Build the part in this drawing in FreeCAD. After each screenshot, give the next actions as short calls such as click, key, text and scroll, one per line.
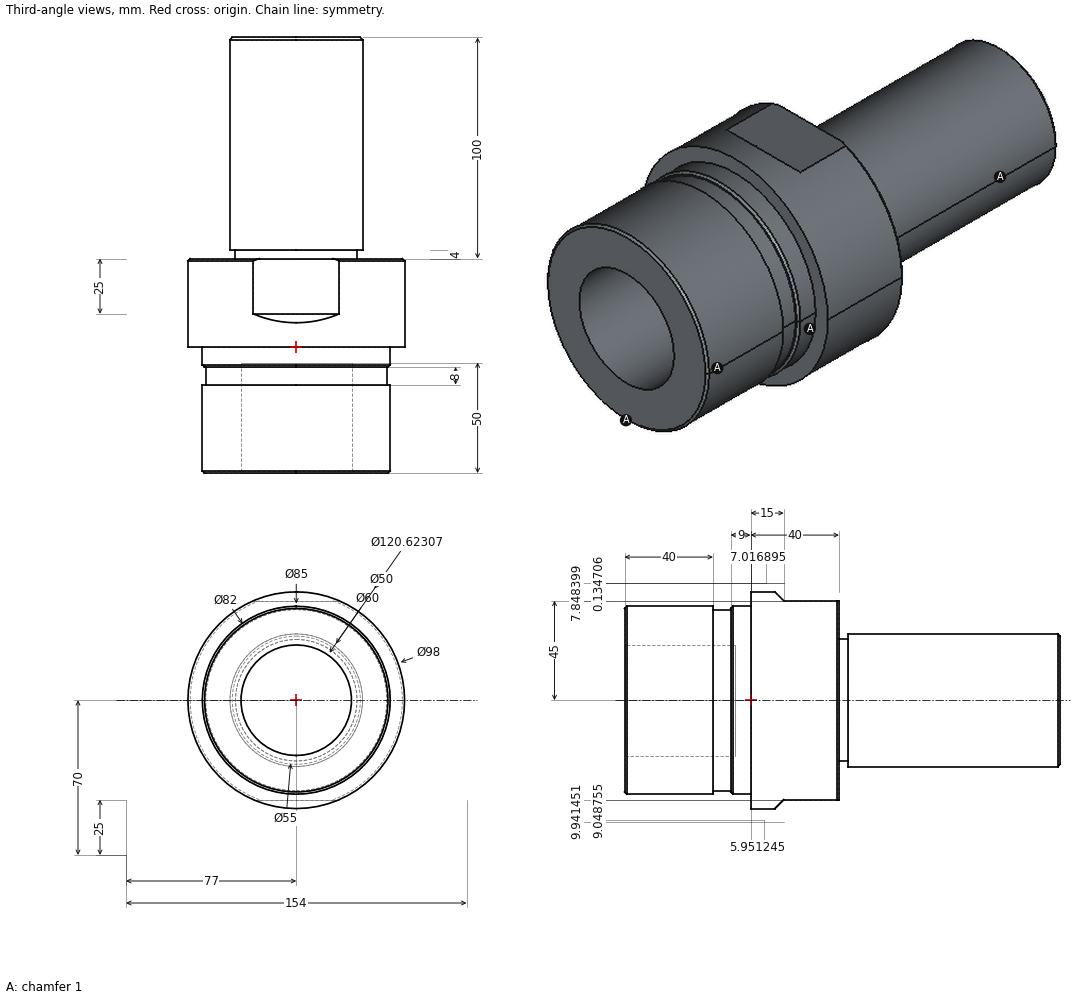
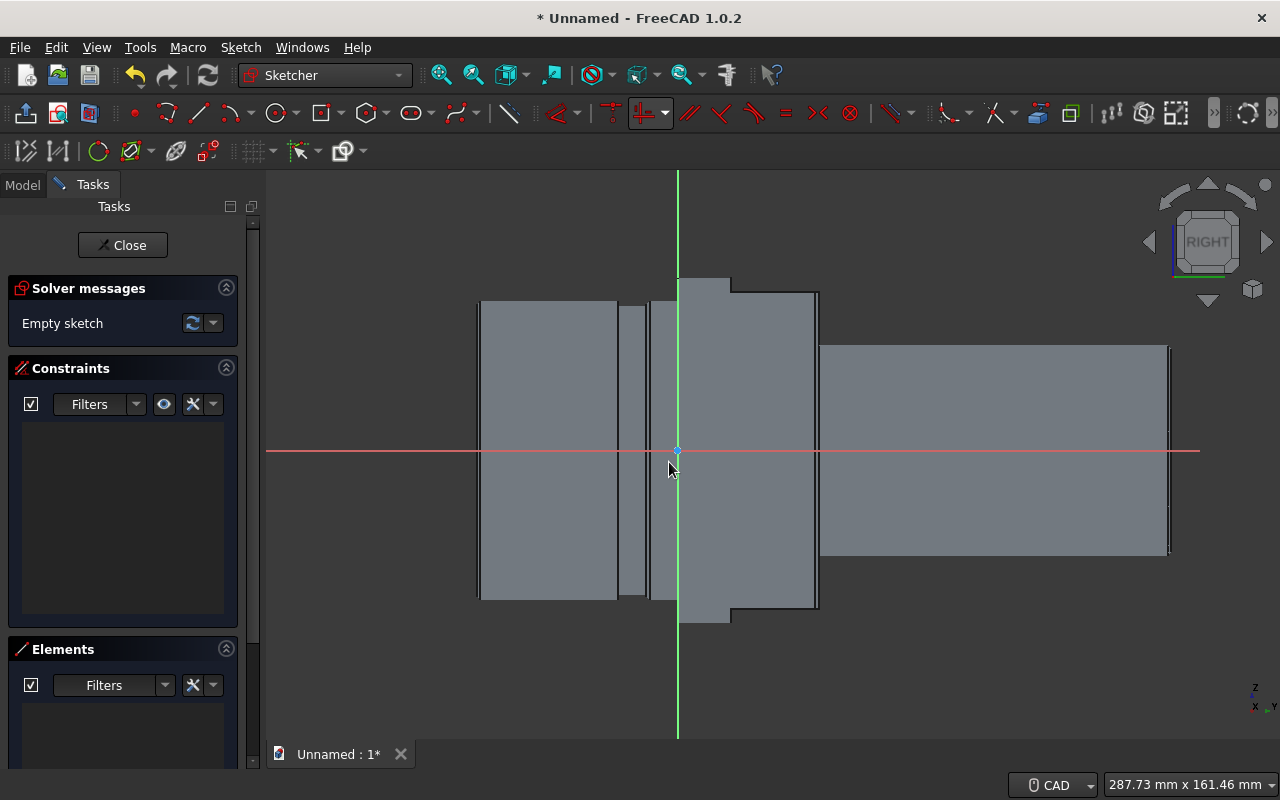
click(168, 114)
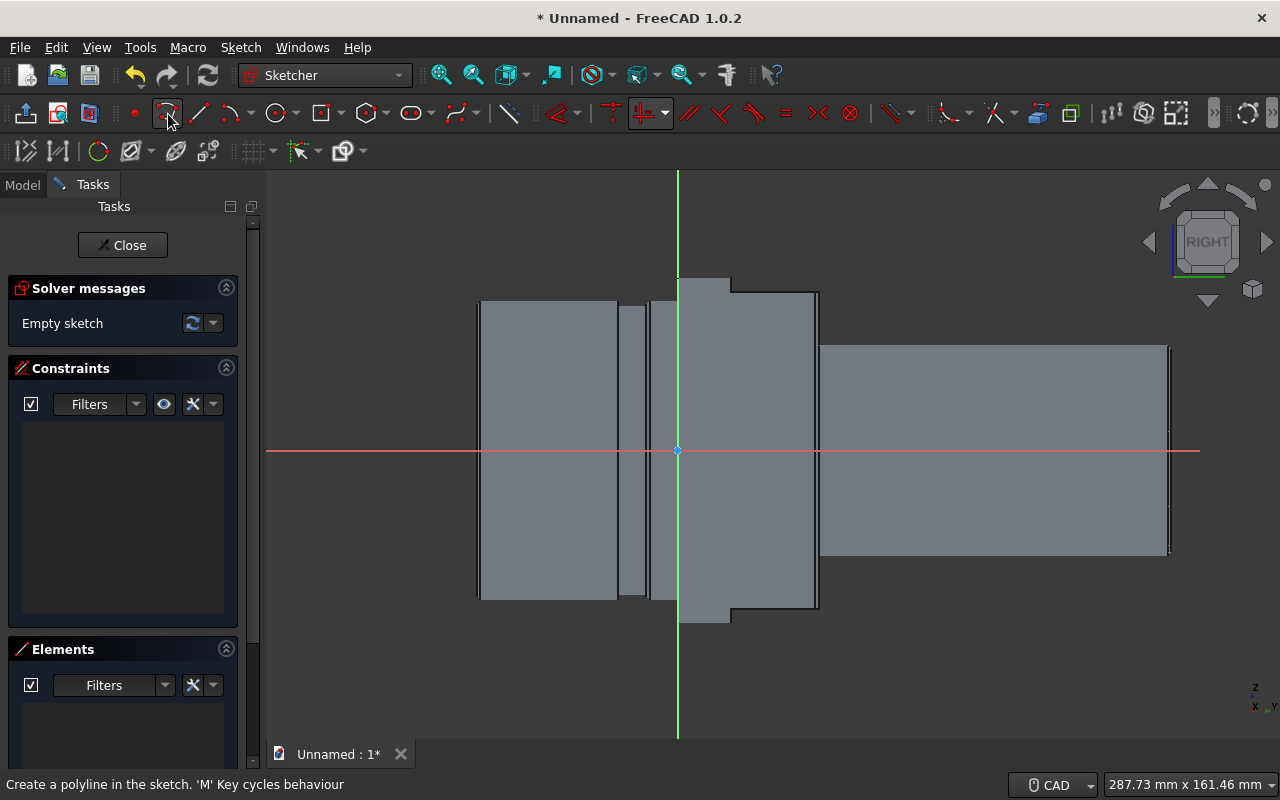
click(731, 292)
click(731, 264)
click(702, 261)
click(731, 293)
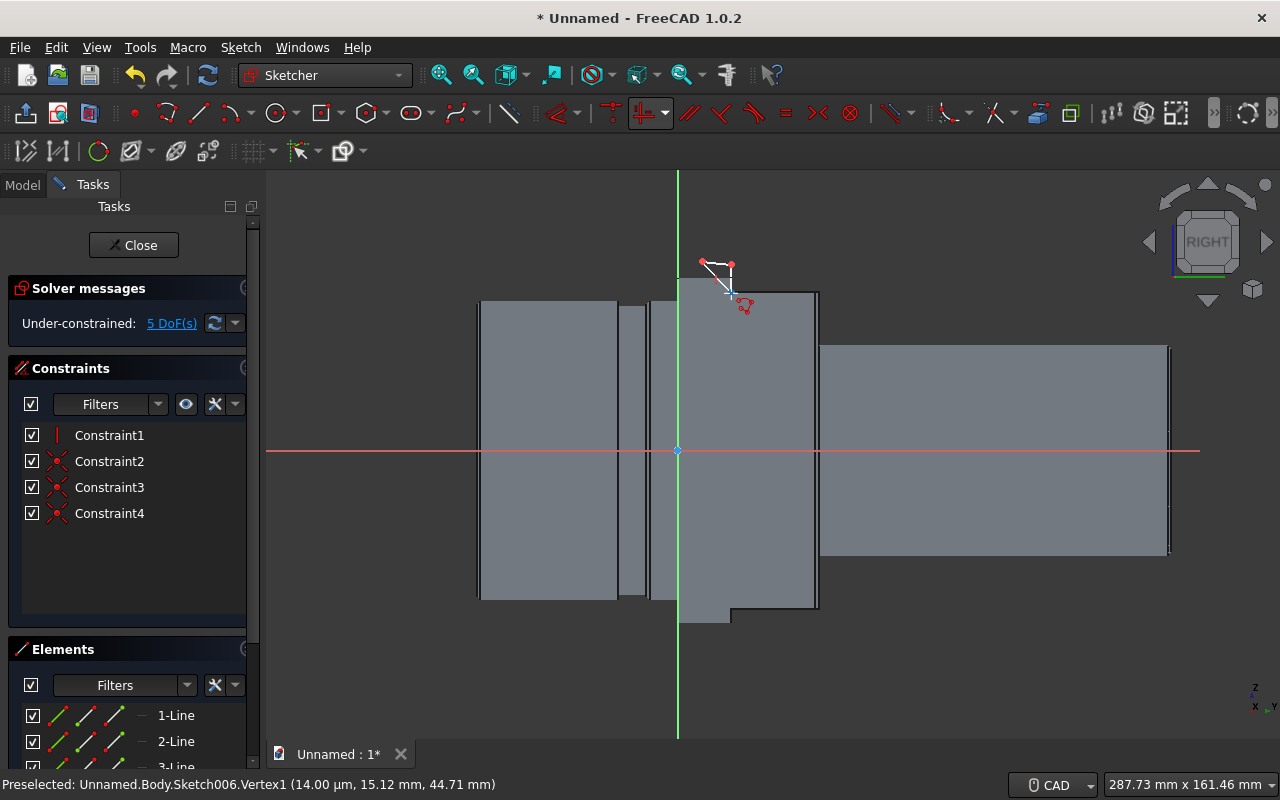
click(731, 609)
click(699, 641)
click(731, 644)
click(731, 610)
key(Escape)
key(Escape)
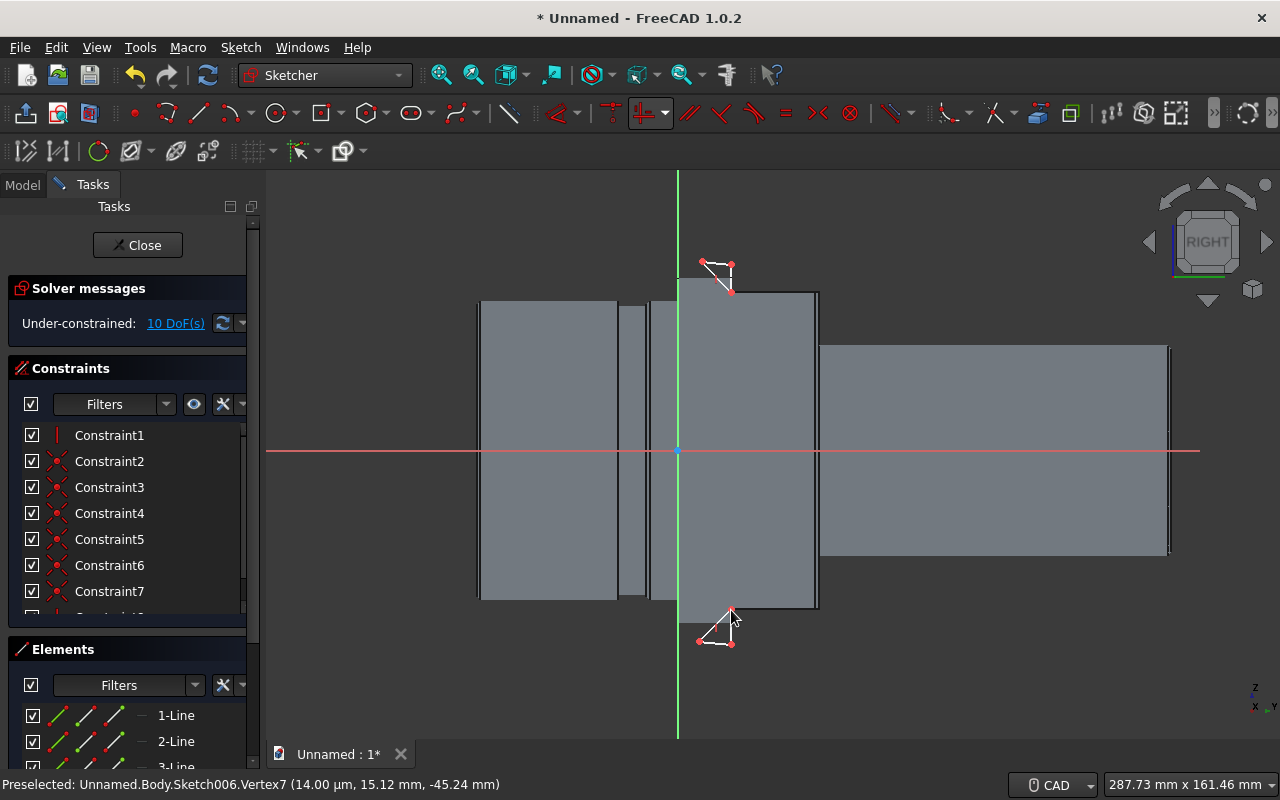
click(731, 293)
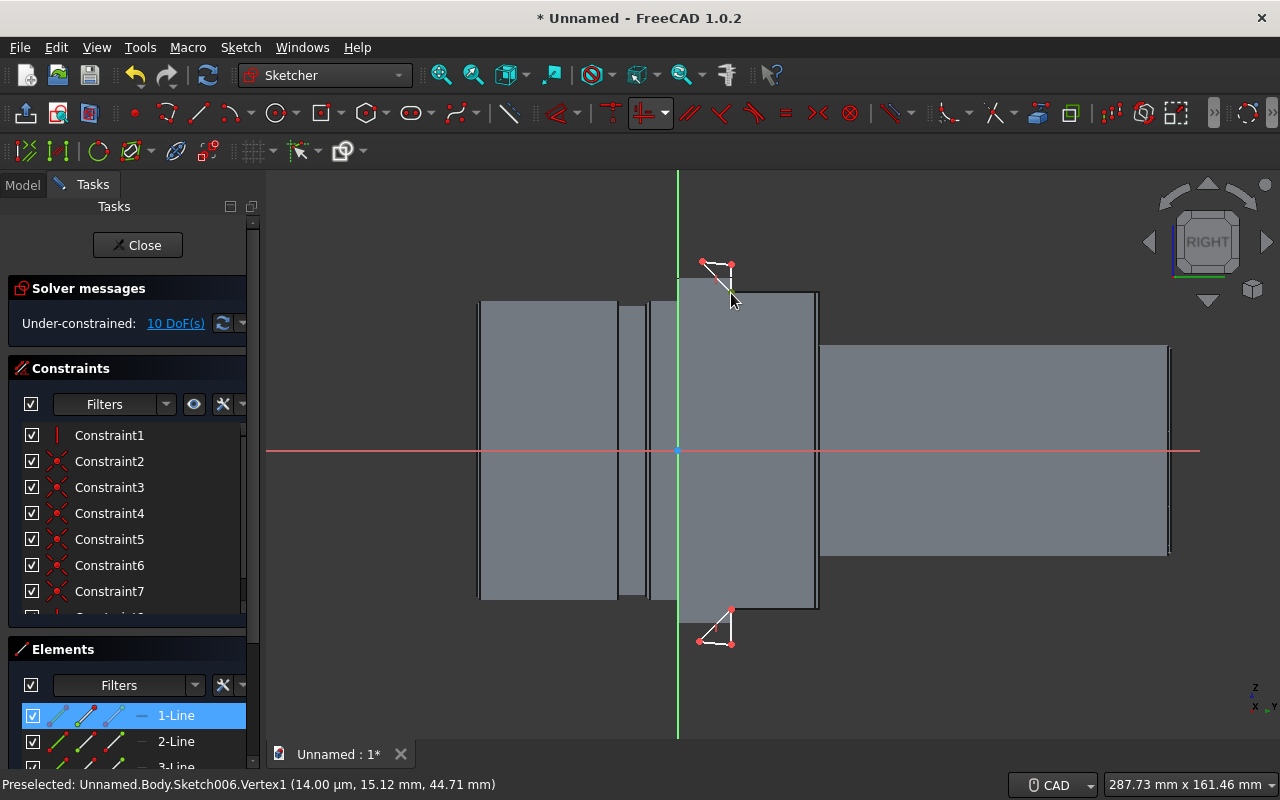
click(731, 610)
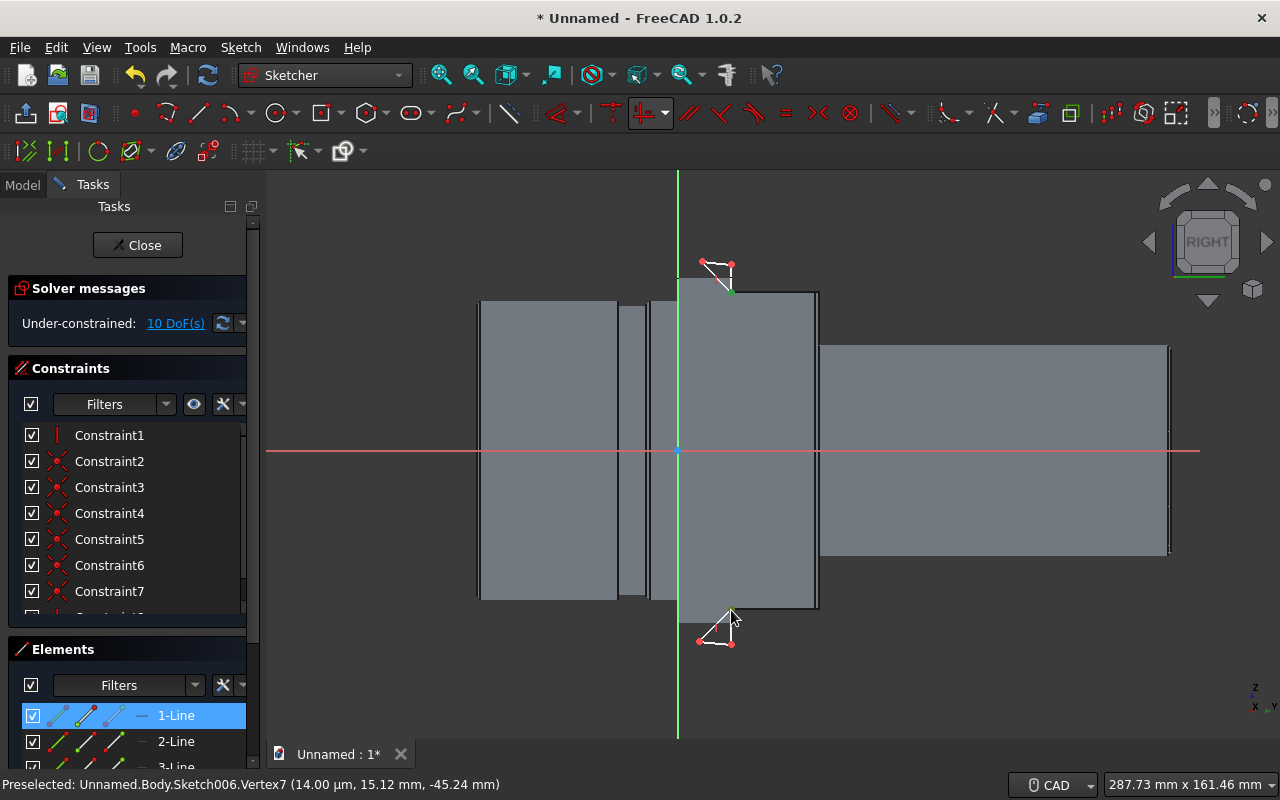
click(353, 451)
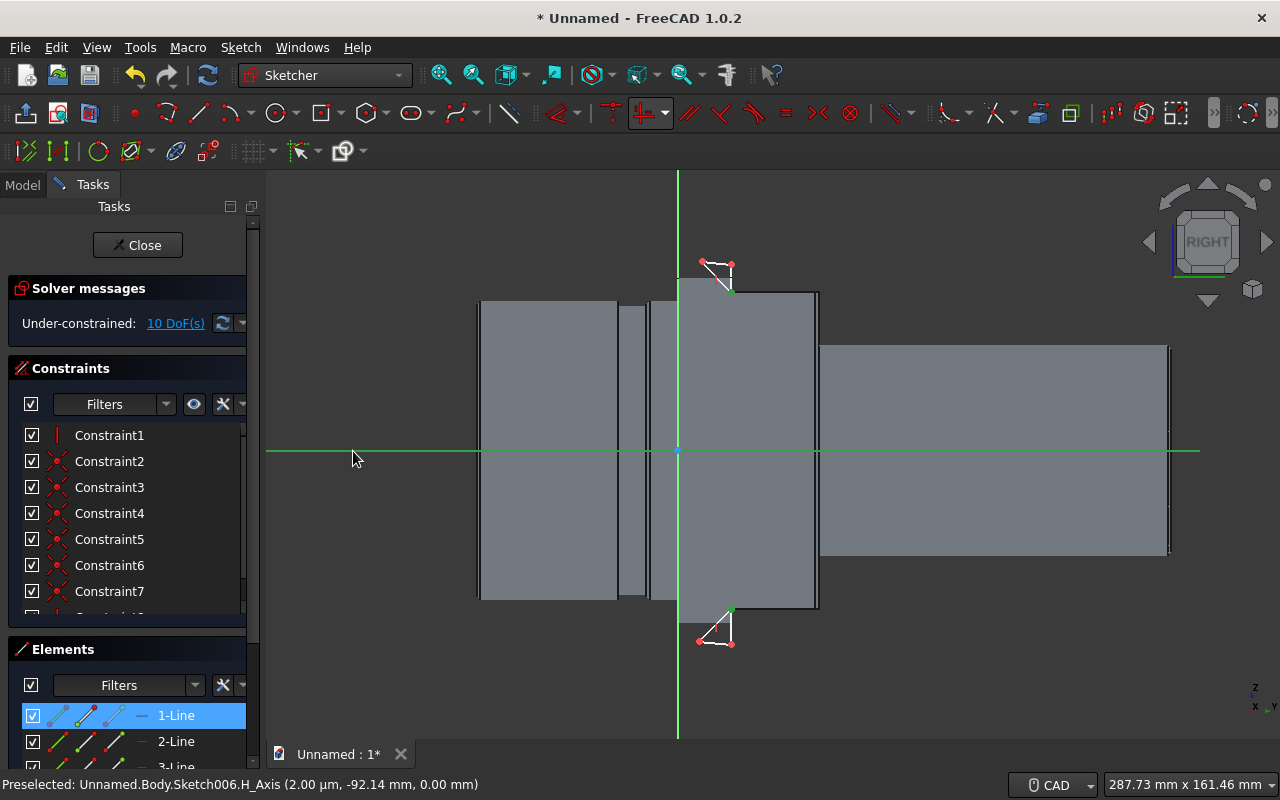
click(818, 114)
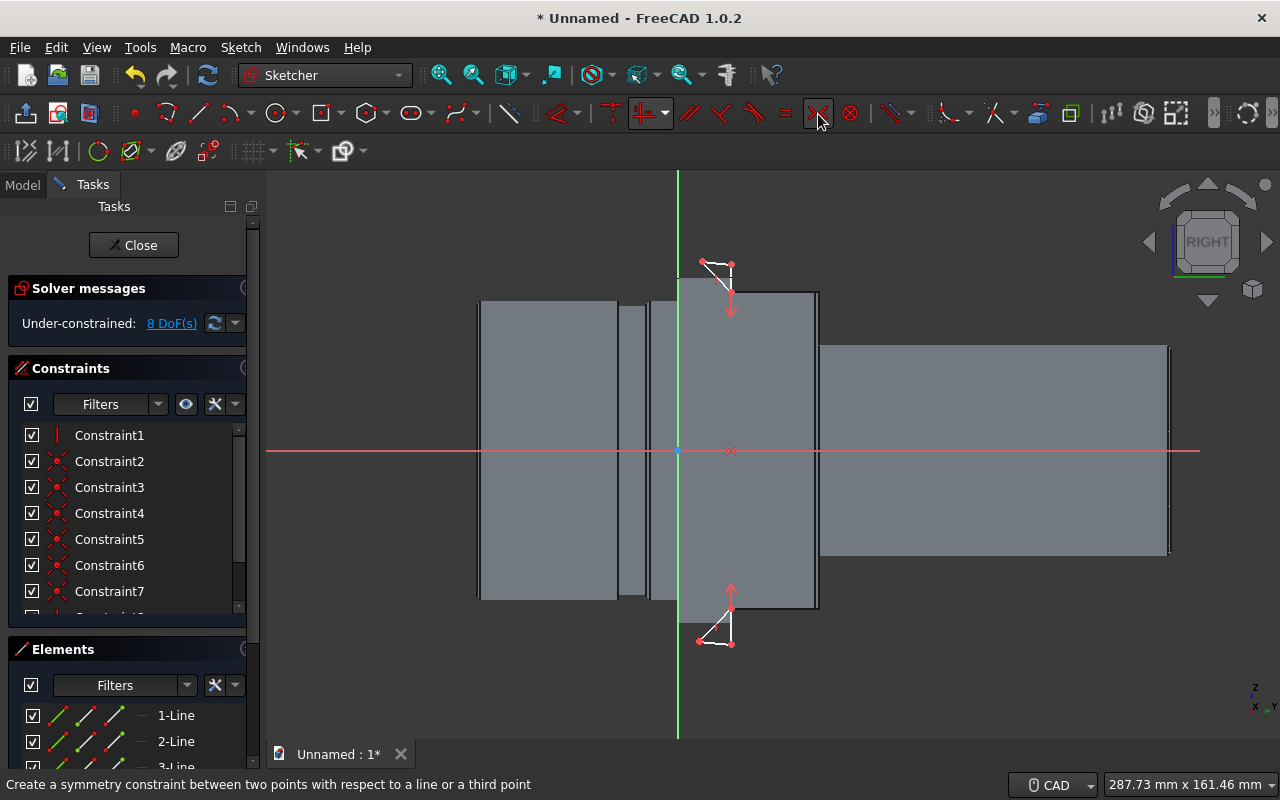
click(556, 114)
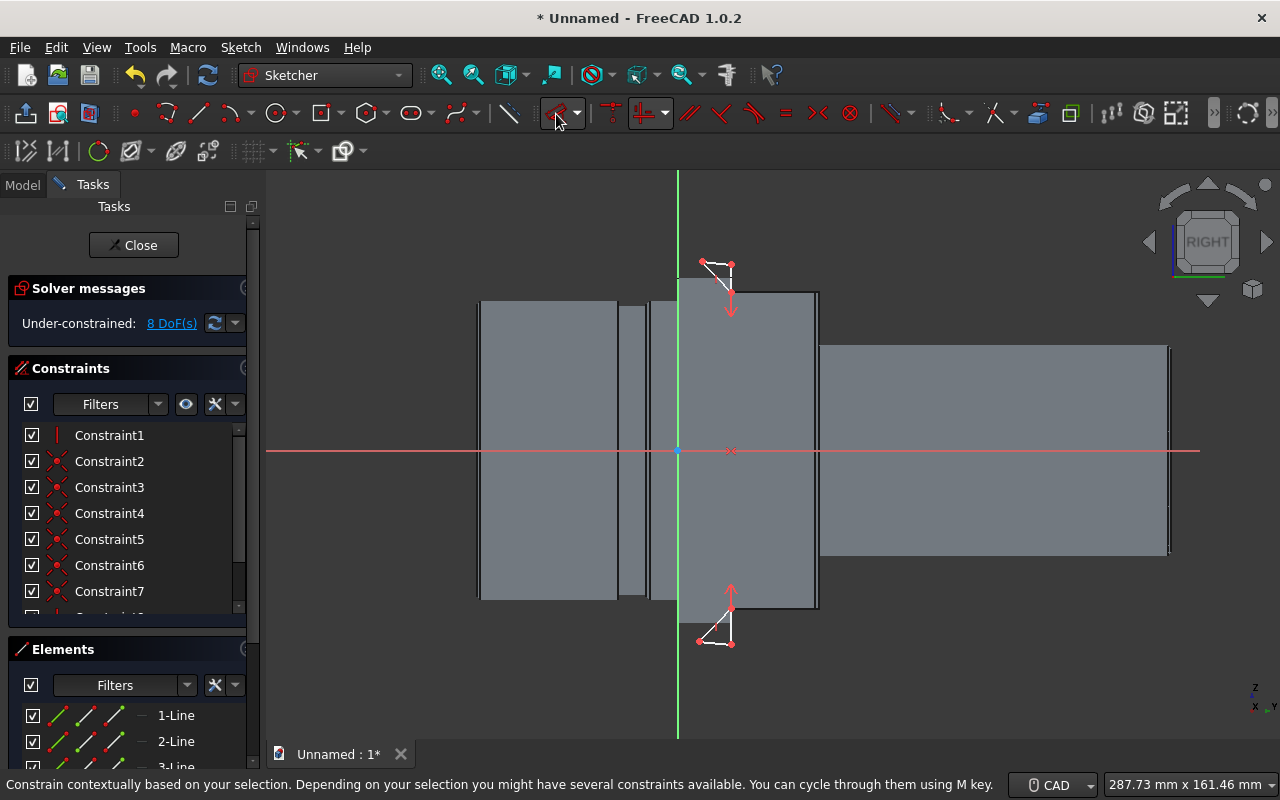
click(731, 292)
click(704, 485)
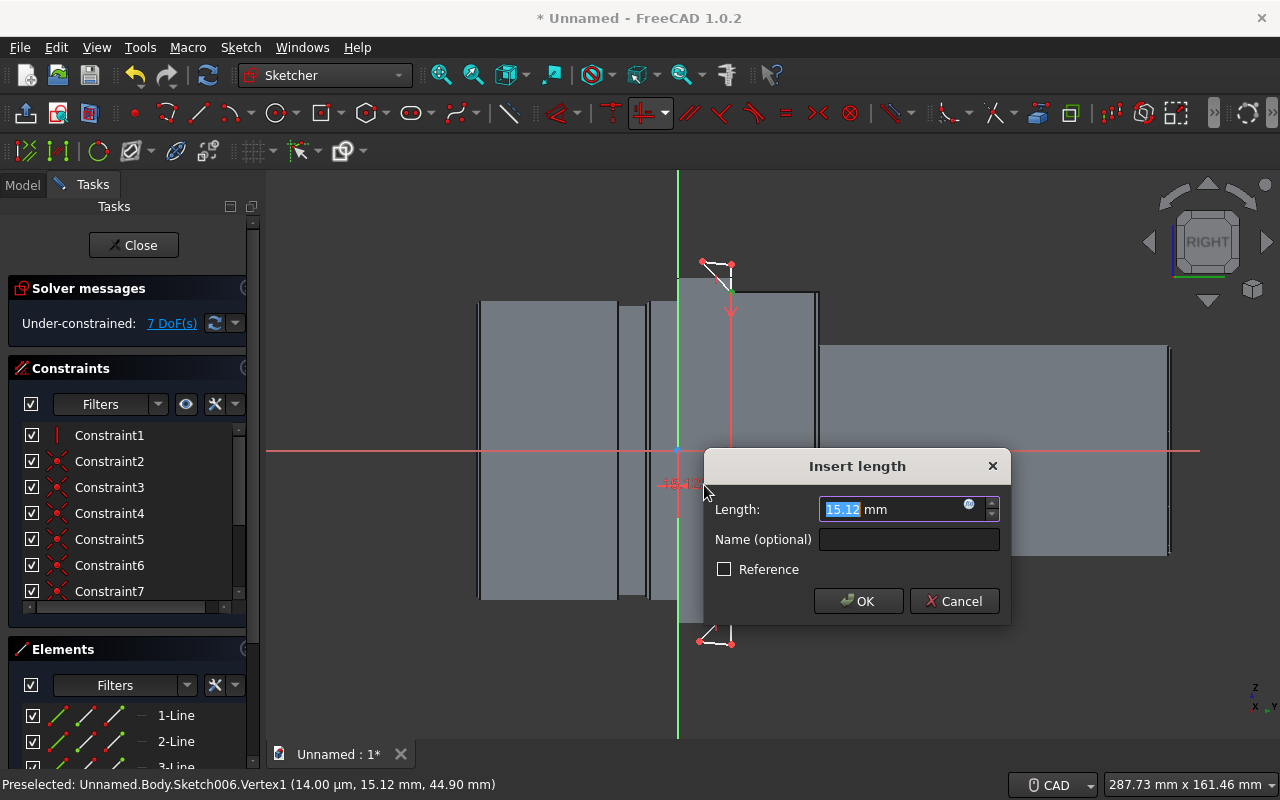
text(15)
key(Return)